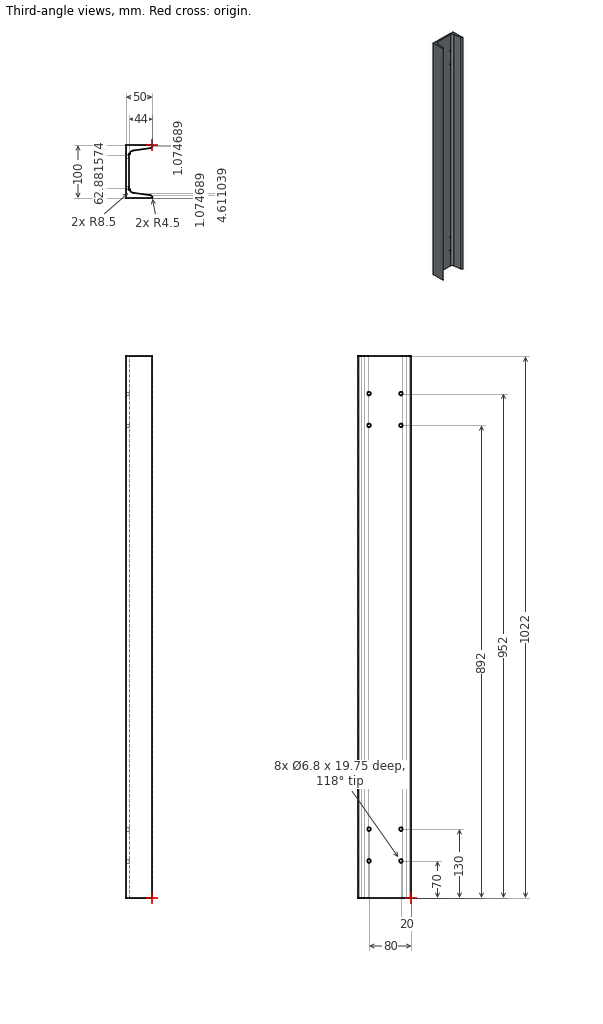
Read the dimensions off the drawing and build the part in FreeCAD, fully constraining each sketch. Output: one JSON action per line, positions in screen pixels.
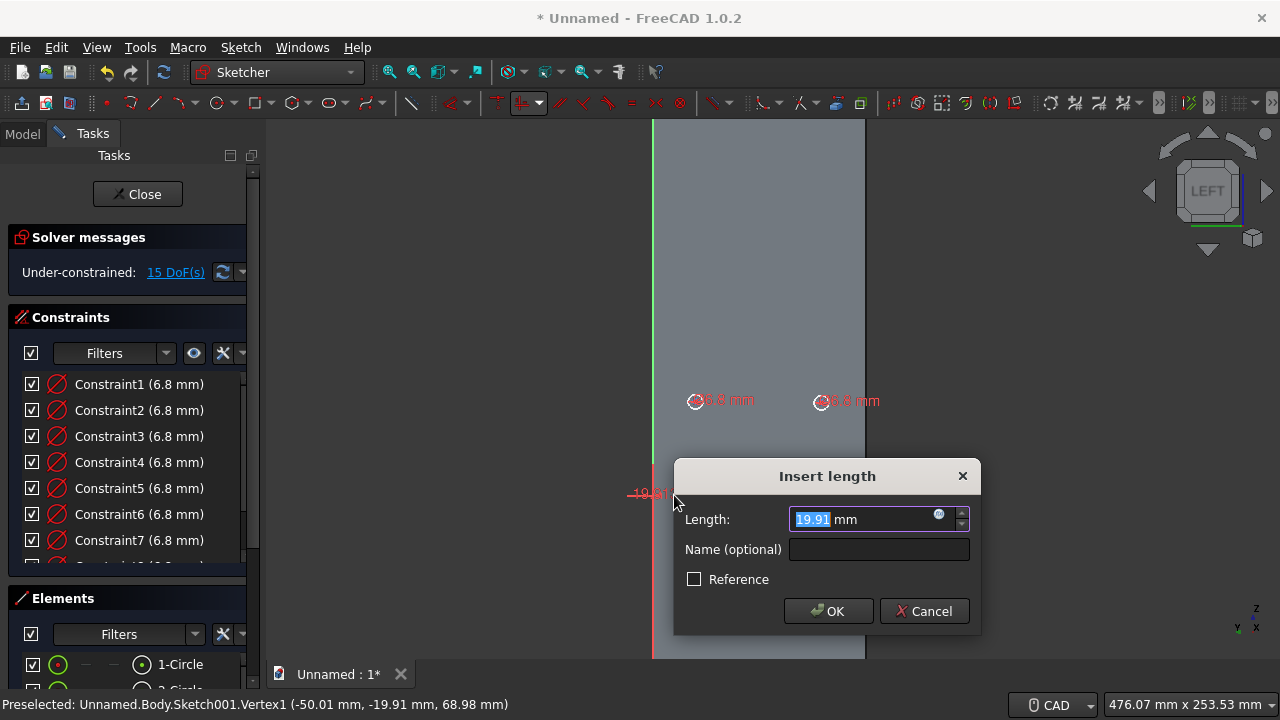
{"action": "type", "text": "20"}
{"action": "key", "text": "Return"}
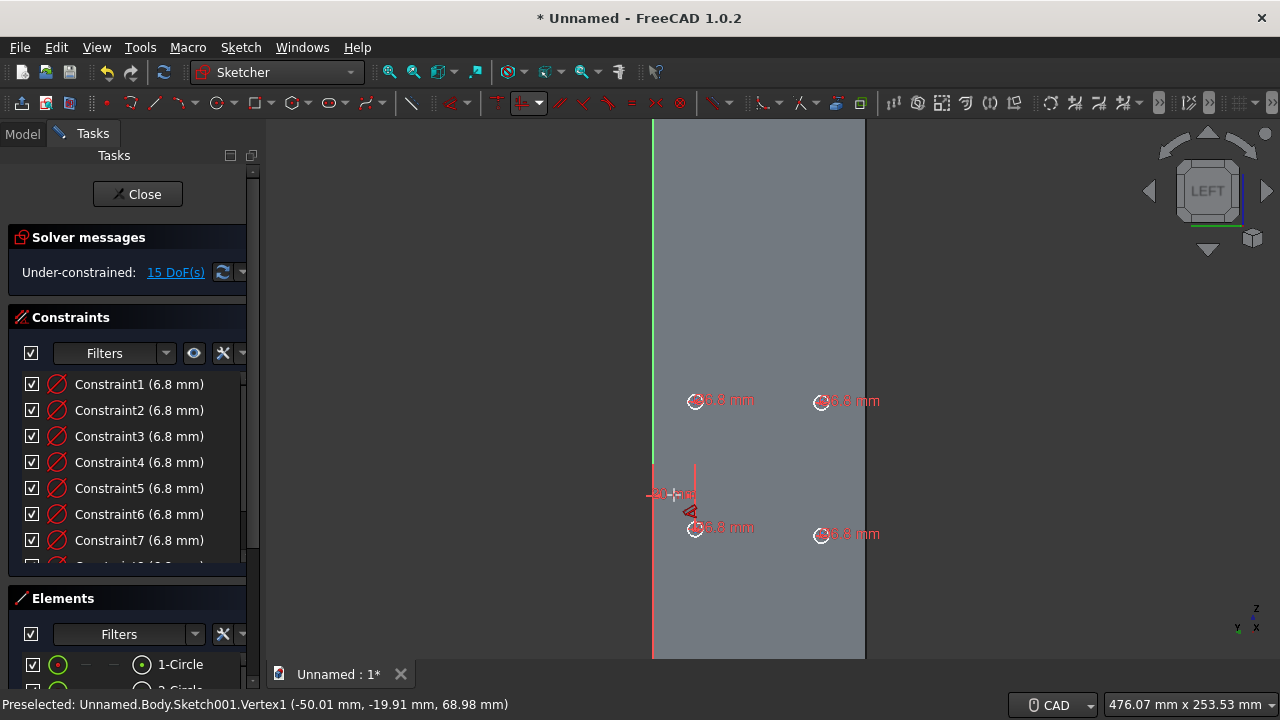
{"action": "scroll", "coordinate": [697, 534], "scroll_direction": "down", "scroll_amount": 9}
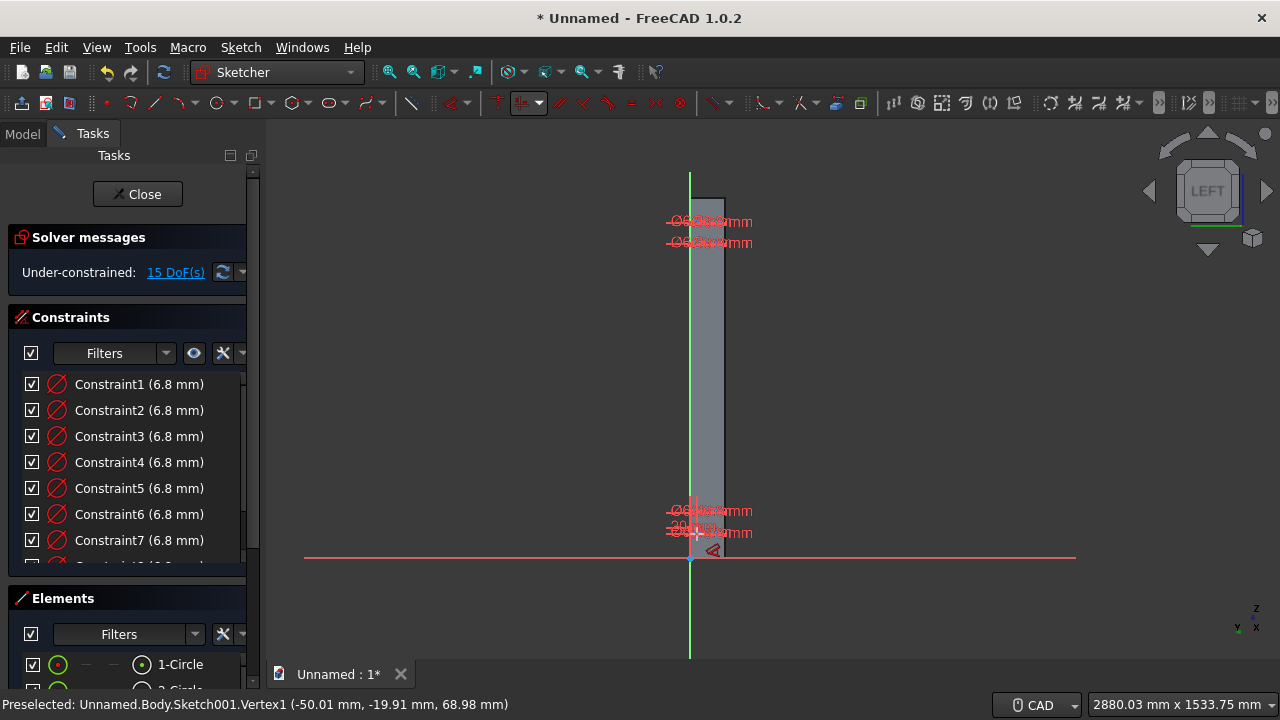
{"action": "scroll", "coordinate": [697, 534], "scroll_direction": "up", "scroll_amount": 3}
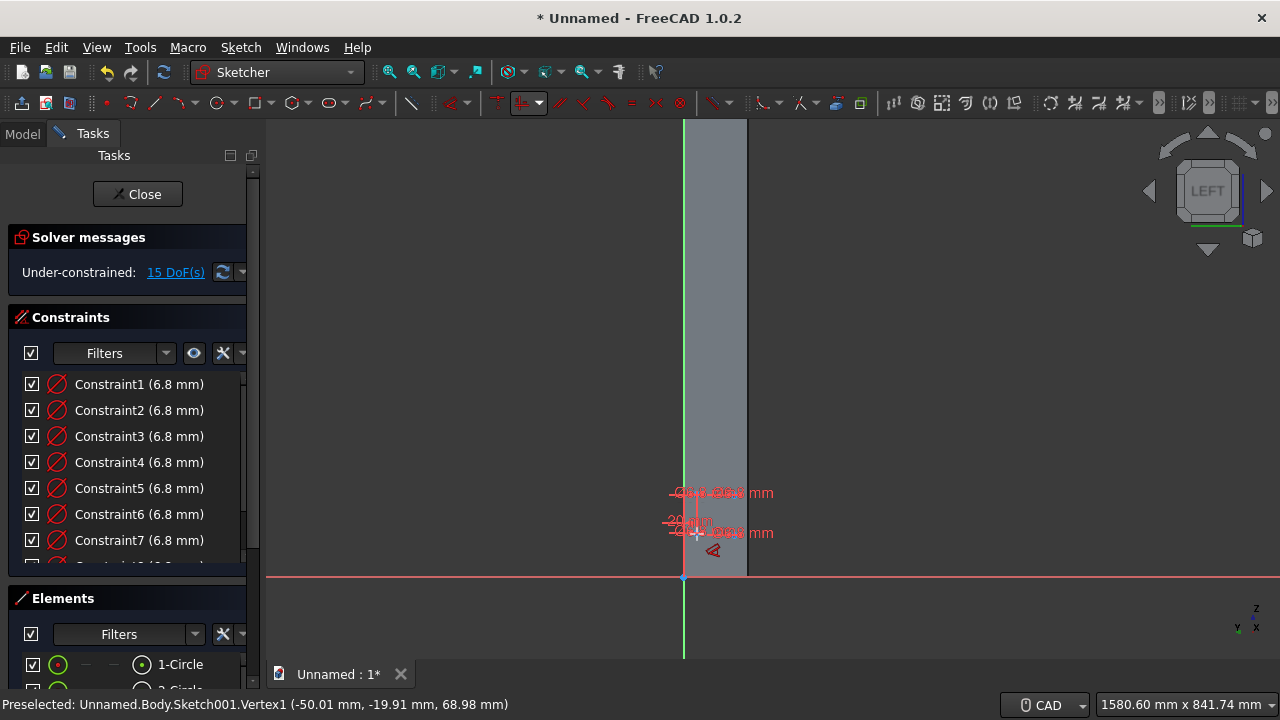
{"action": "left_click", "coordinate": [697, 533]}
{"action": "left_click", "coordinate": [650, 555]}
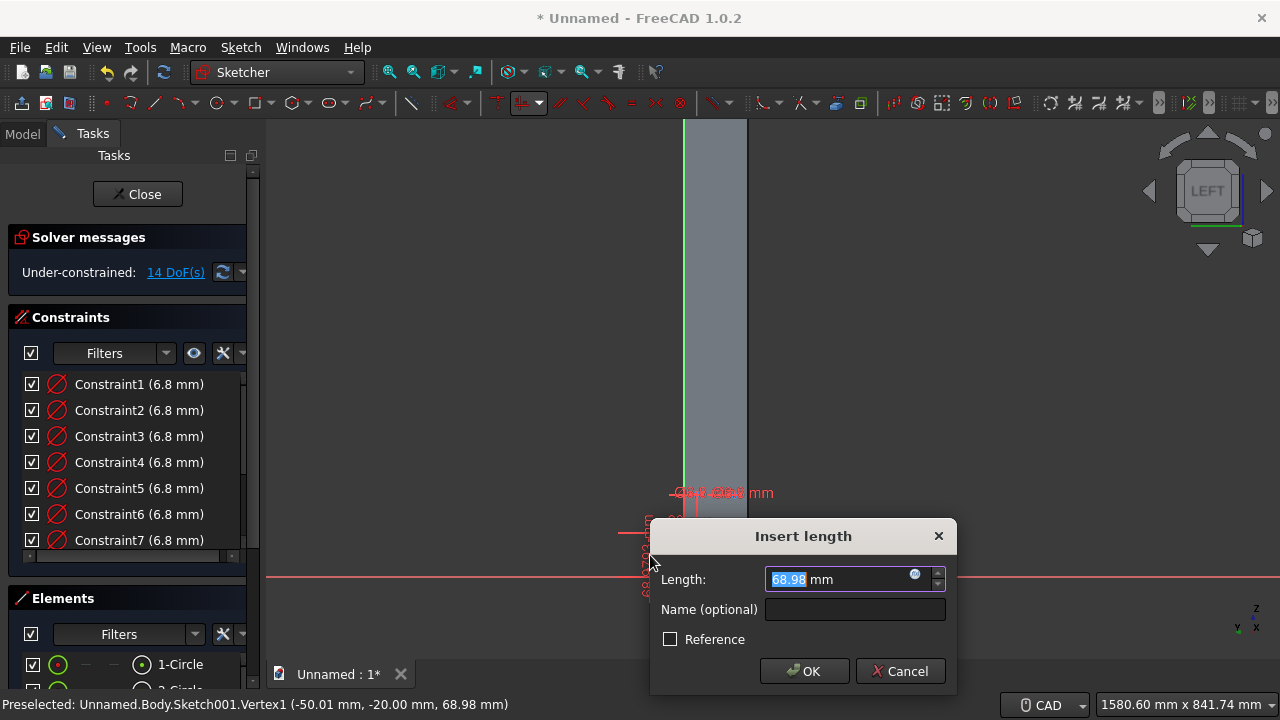
{"action": "type", "text": "70"}
{"action": "key", "text": "Return"}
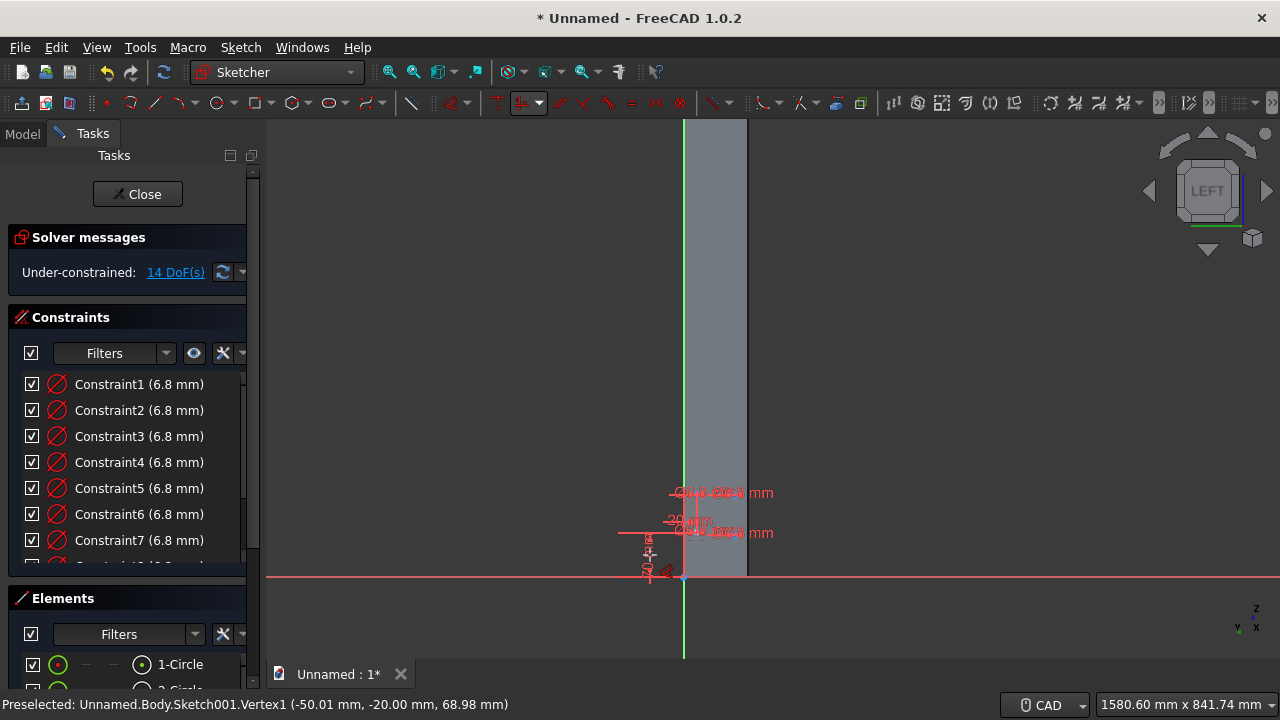
{"action": "scroll", "coordinate": [697, 495], "scroll_direction": "up", "scroll_amount": 6}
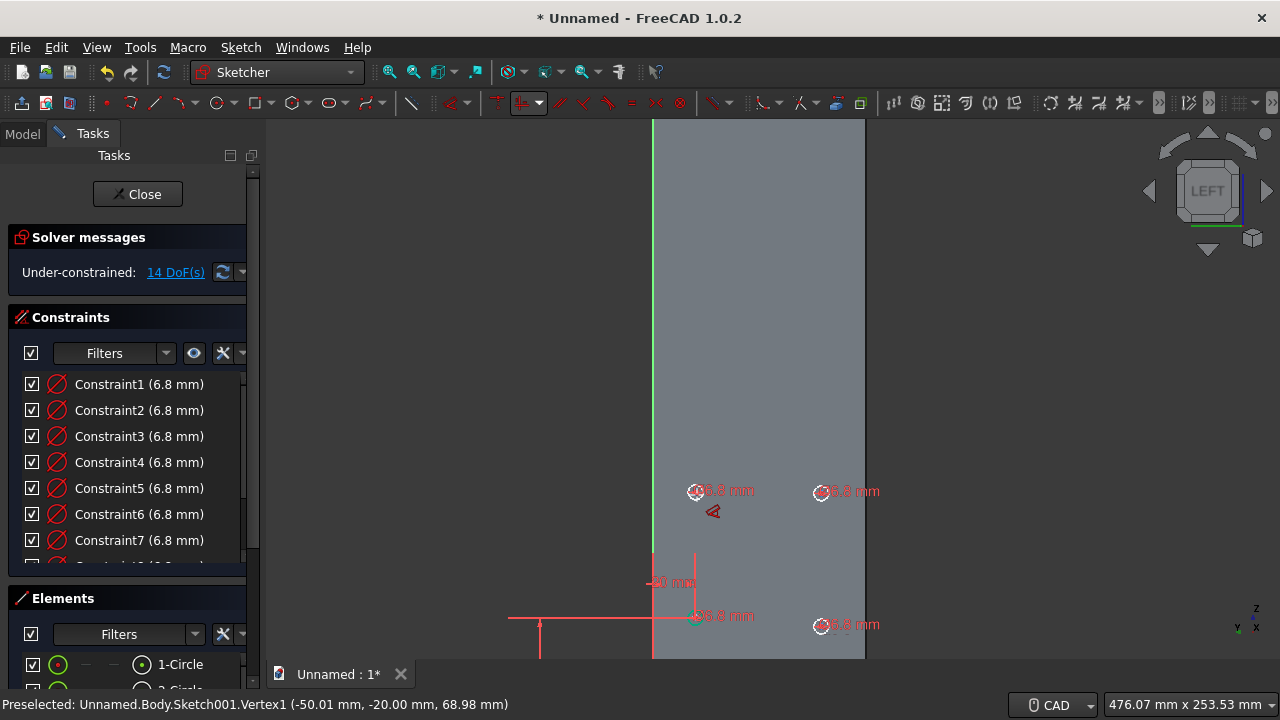
{"action": "left_click", "coordinate": [696, 492]}
{"action": "left_click", "coordinate": [674, 458]}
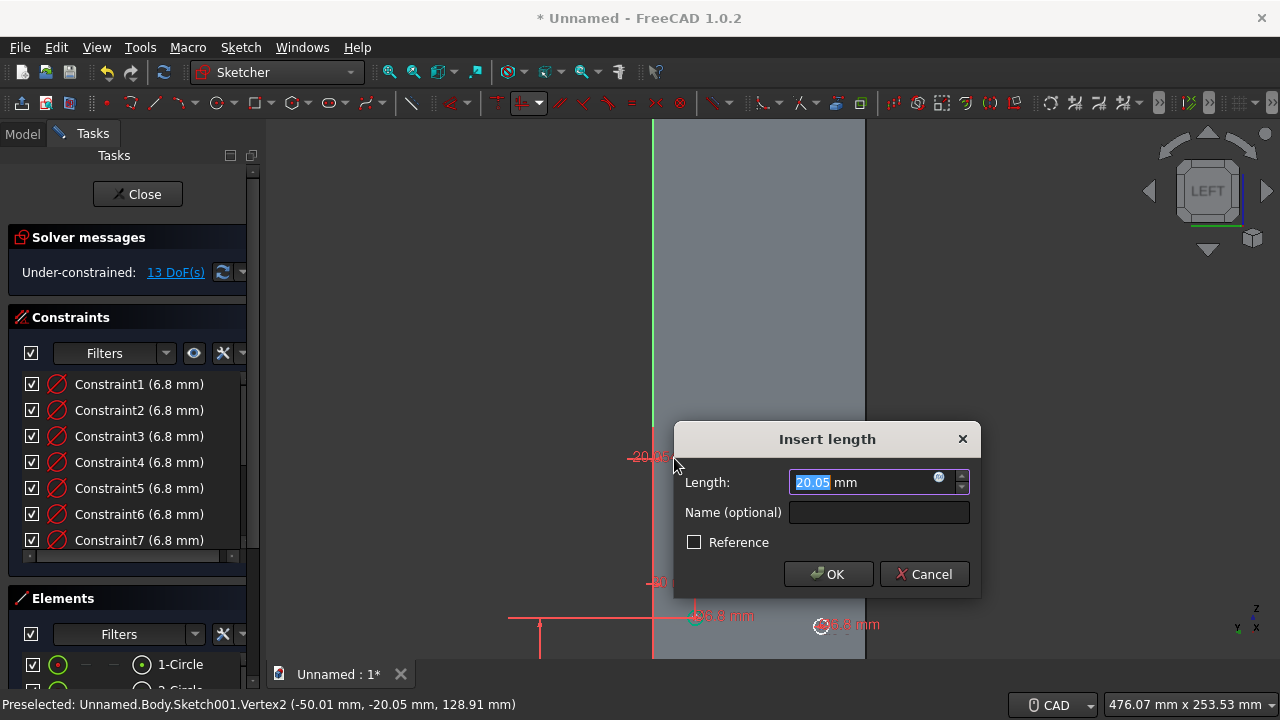
{"action": "type", "text": "20"}
{"action": "key", "text": "Return"}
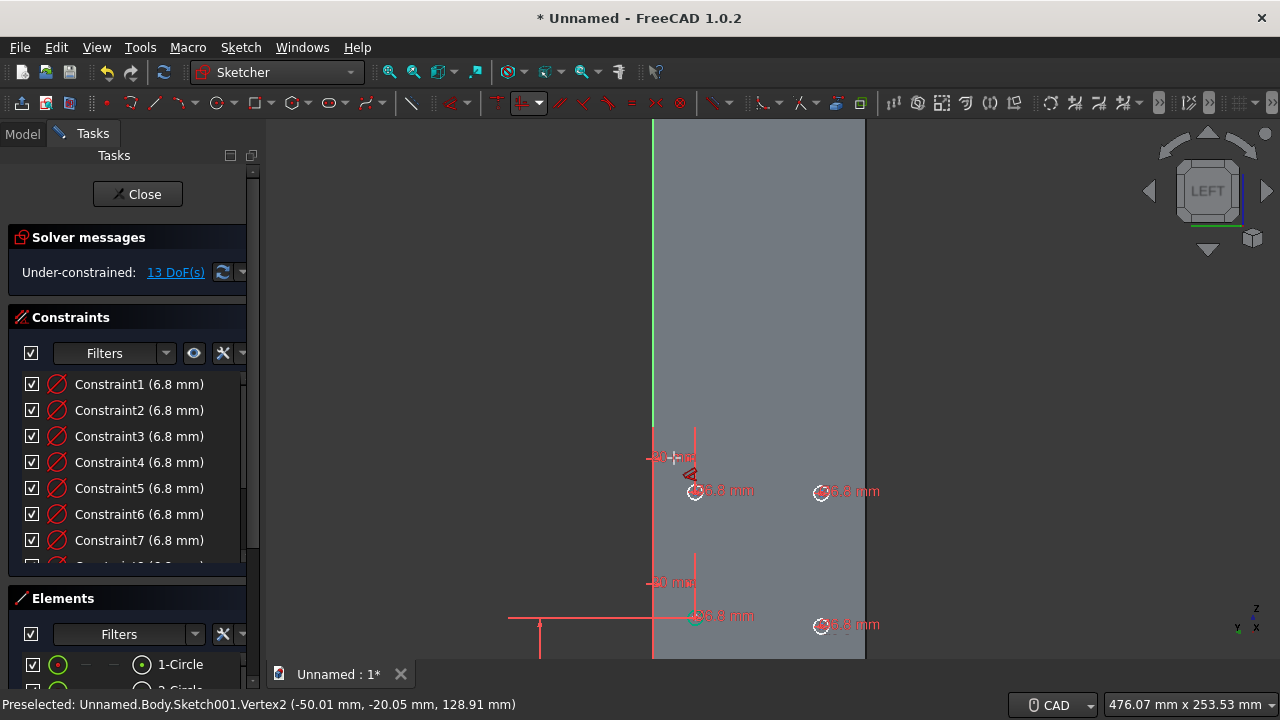
{"action": "scroll", "coordinate": [697, 516], "scroll_direction": "down", "scroll_amount": 9}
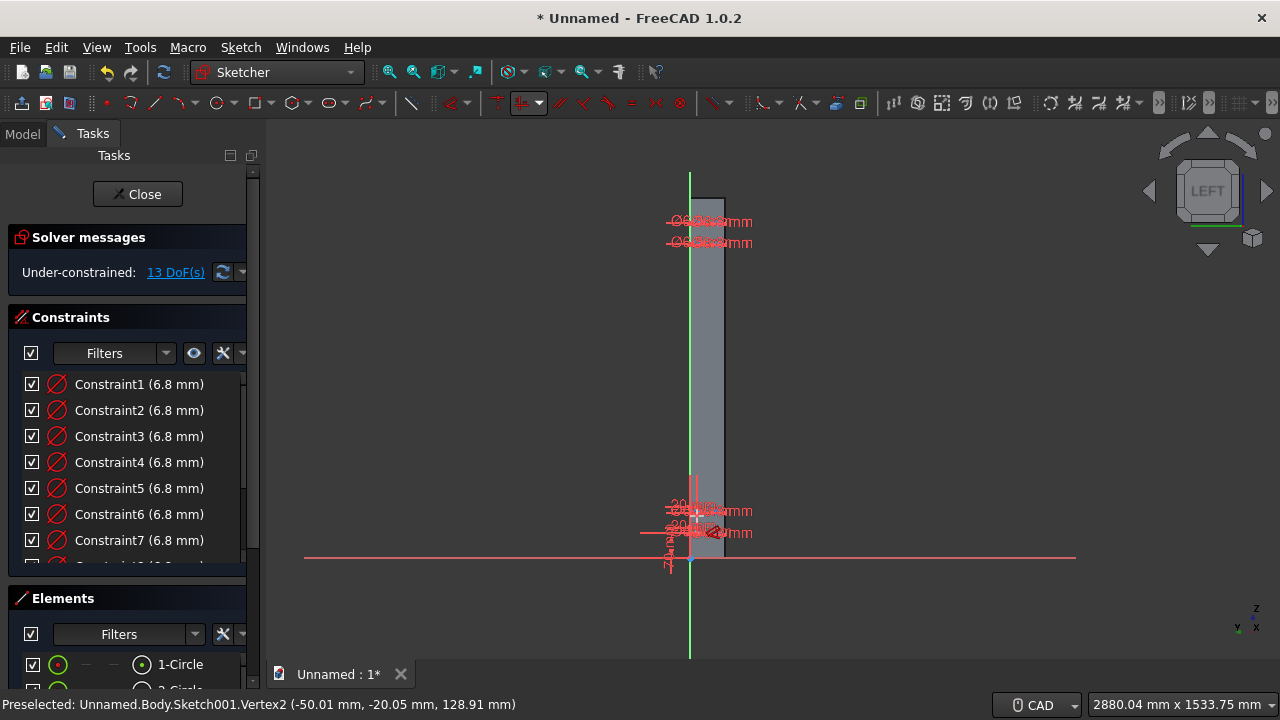
{"action": "scroll", "coordinate": [718, 513], "scroll_direction": "up", "scroll_amount": 2}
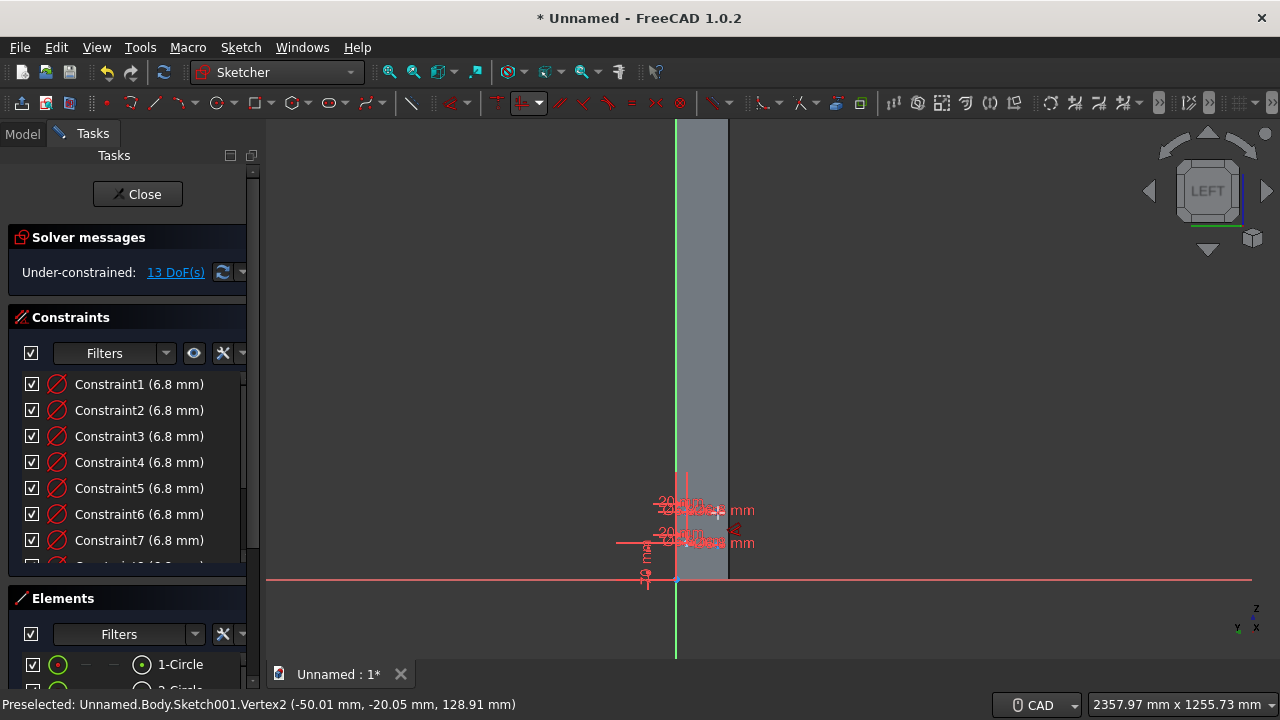
{"action": "left_click", "coordinate": [718, 512]}
{"action": "left_click", "coordinate": [697, 614]}